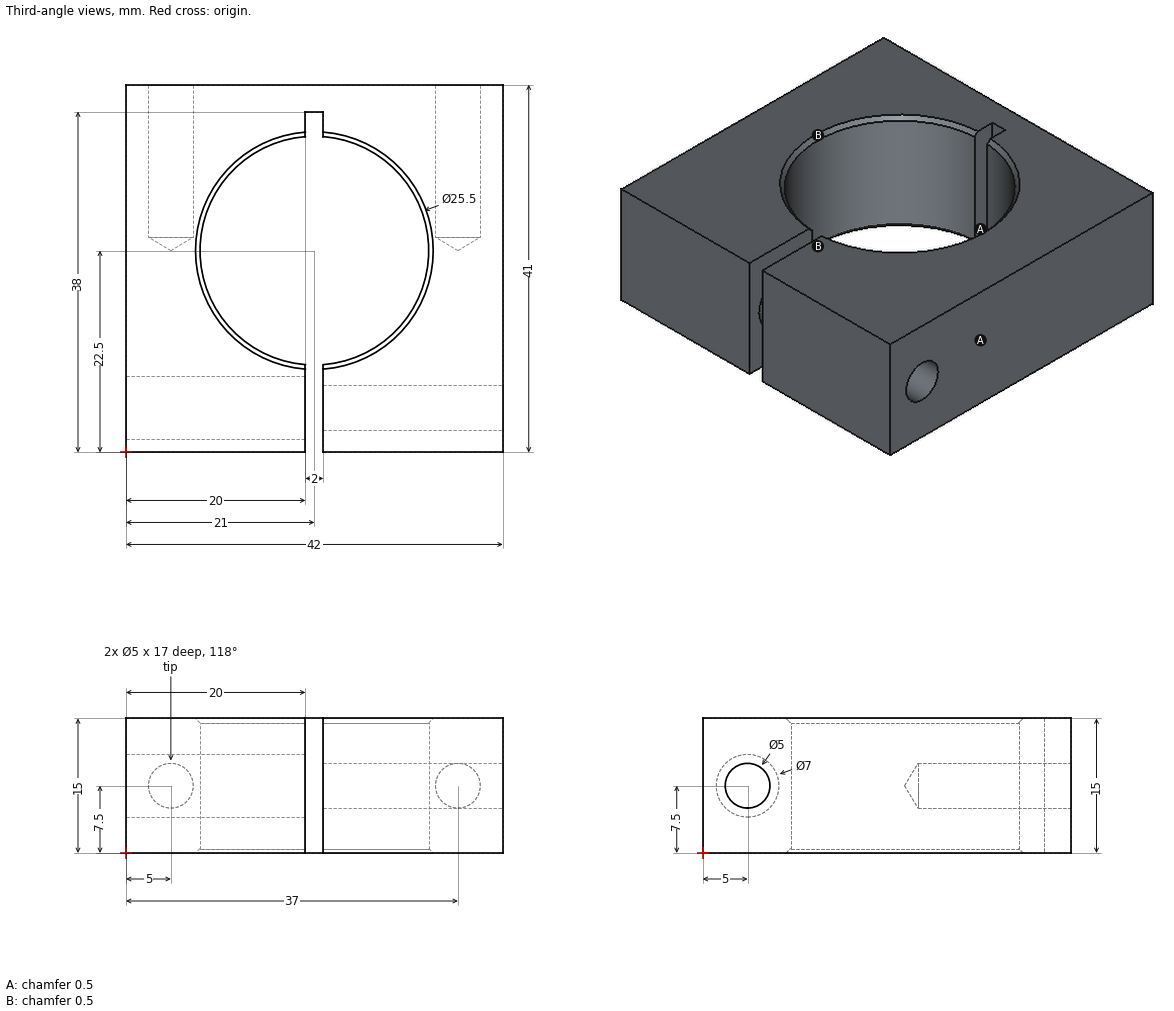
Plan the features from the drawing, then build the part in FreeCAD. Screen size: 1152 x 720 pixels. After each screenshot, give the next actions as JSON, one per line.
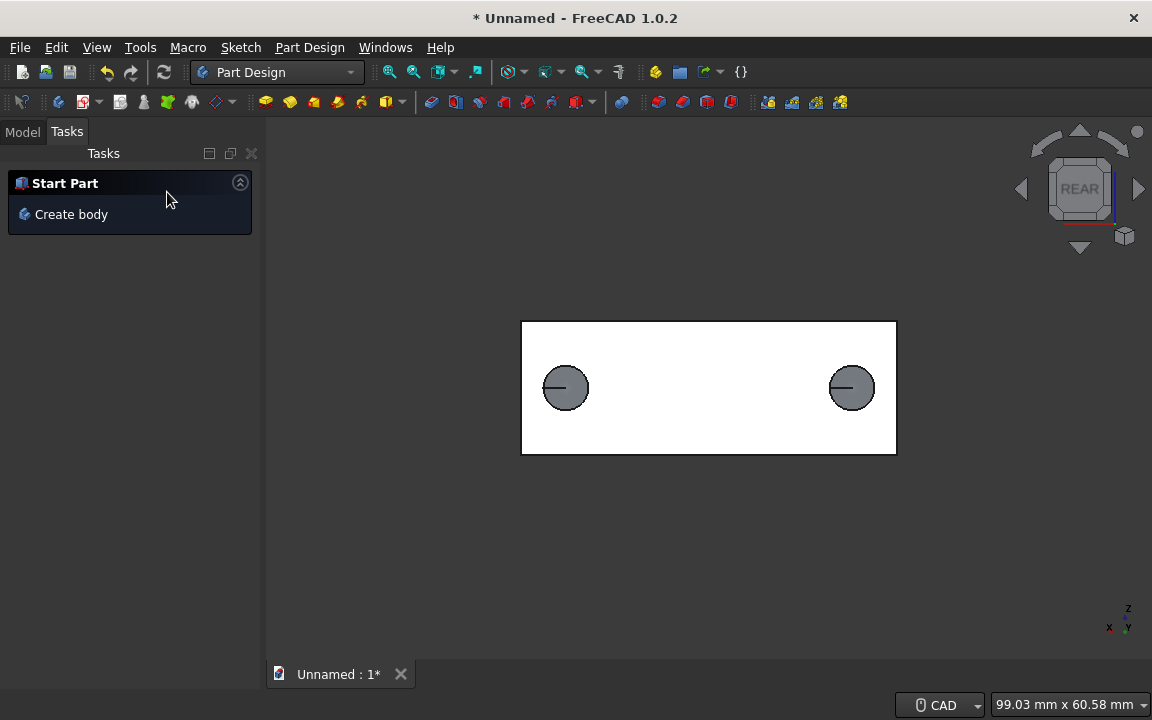
{"action": "left_click", "coordinate": [390, 72]}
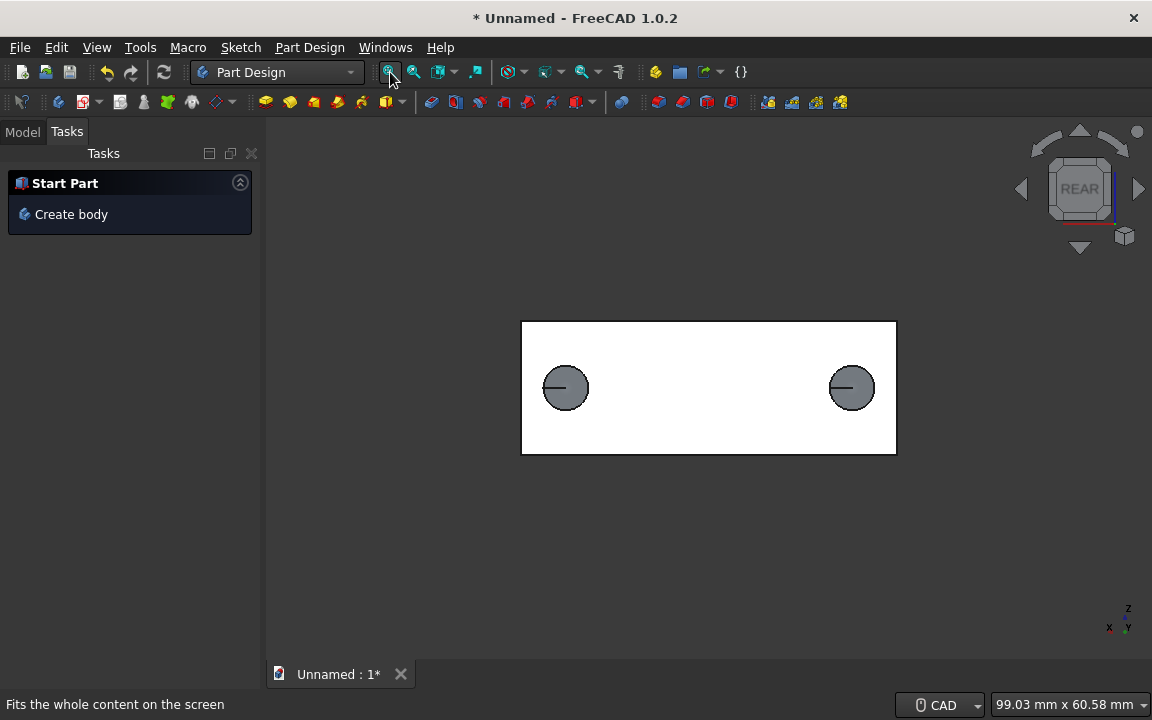
{"action": "key", "text": "6"}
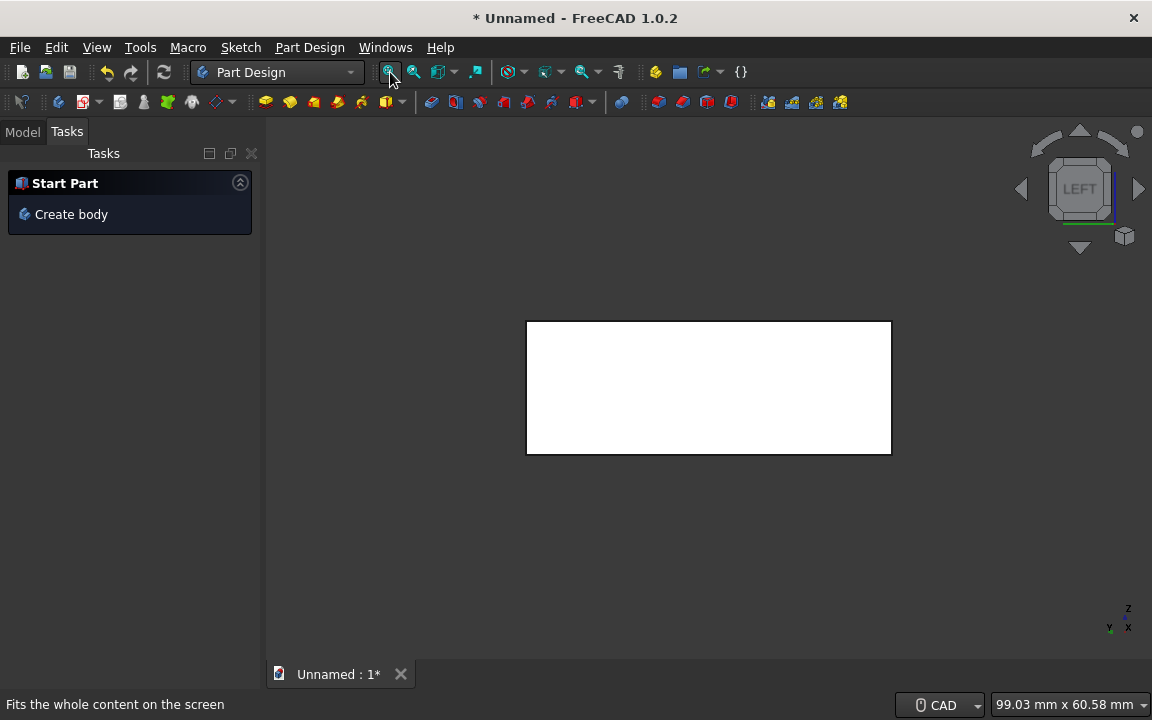
{"action": "left_click", "coordinate": [390, 72]}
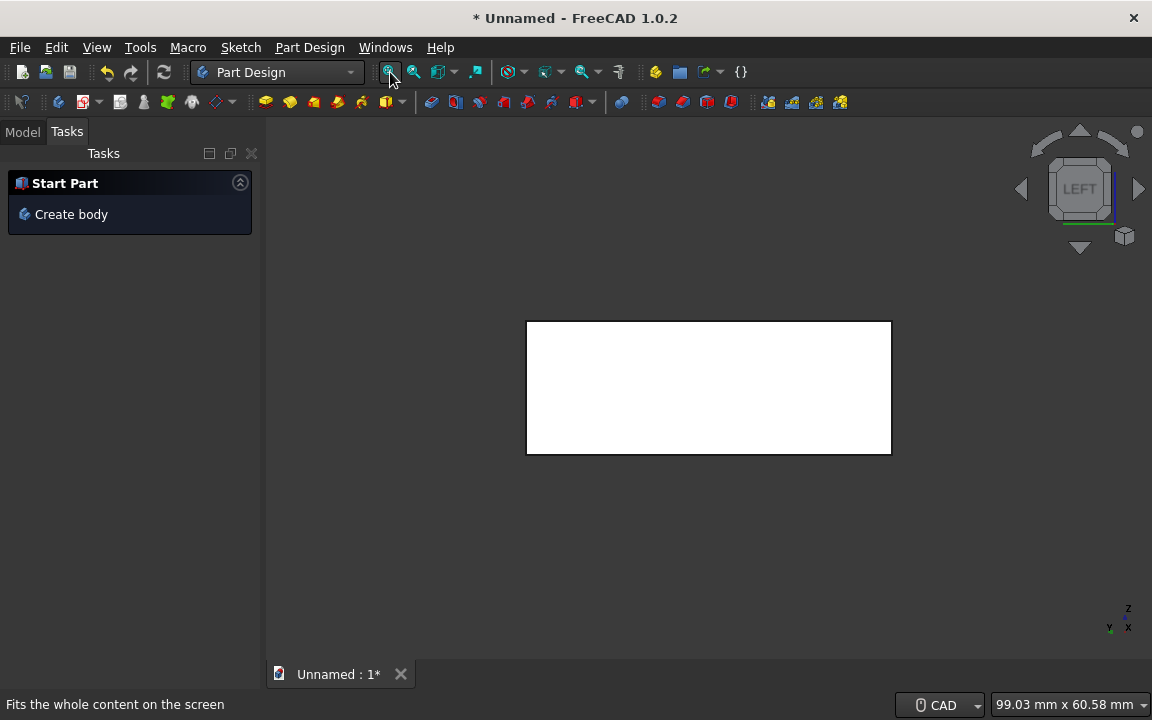
{"action": "left_click", "coordinate": [604, 387]}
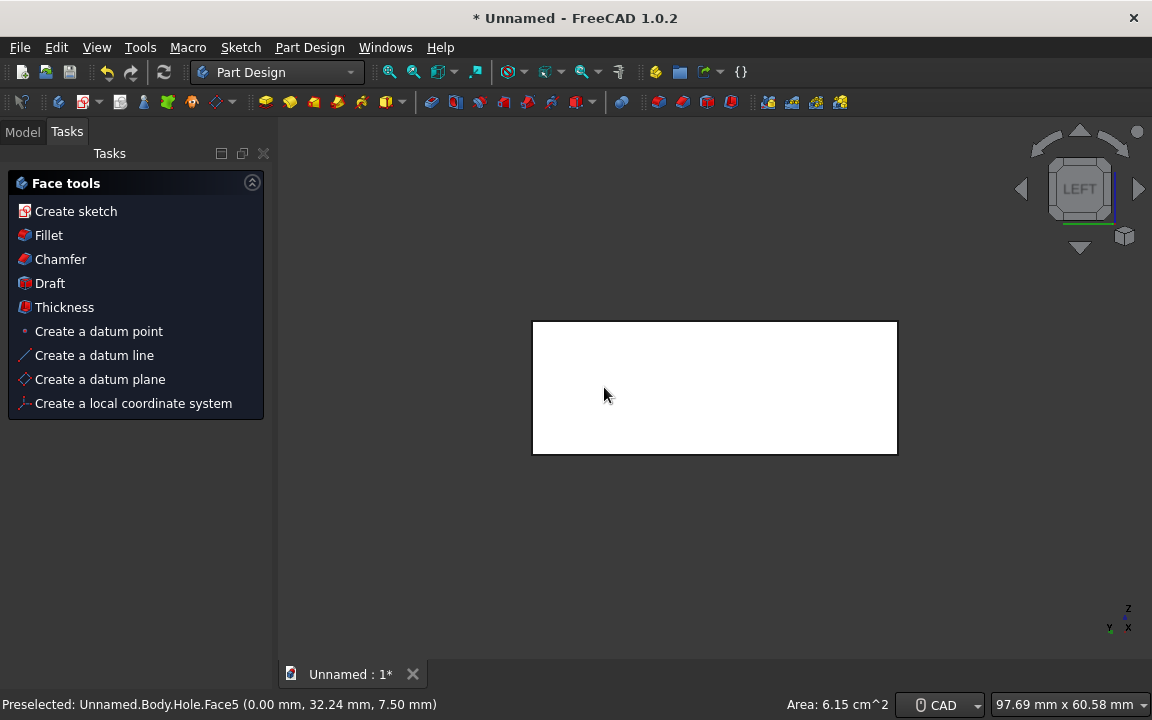
{"action": "left_click", "coordinate": [84, 102]}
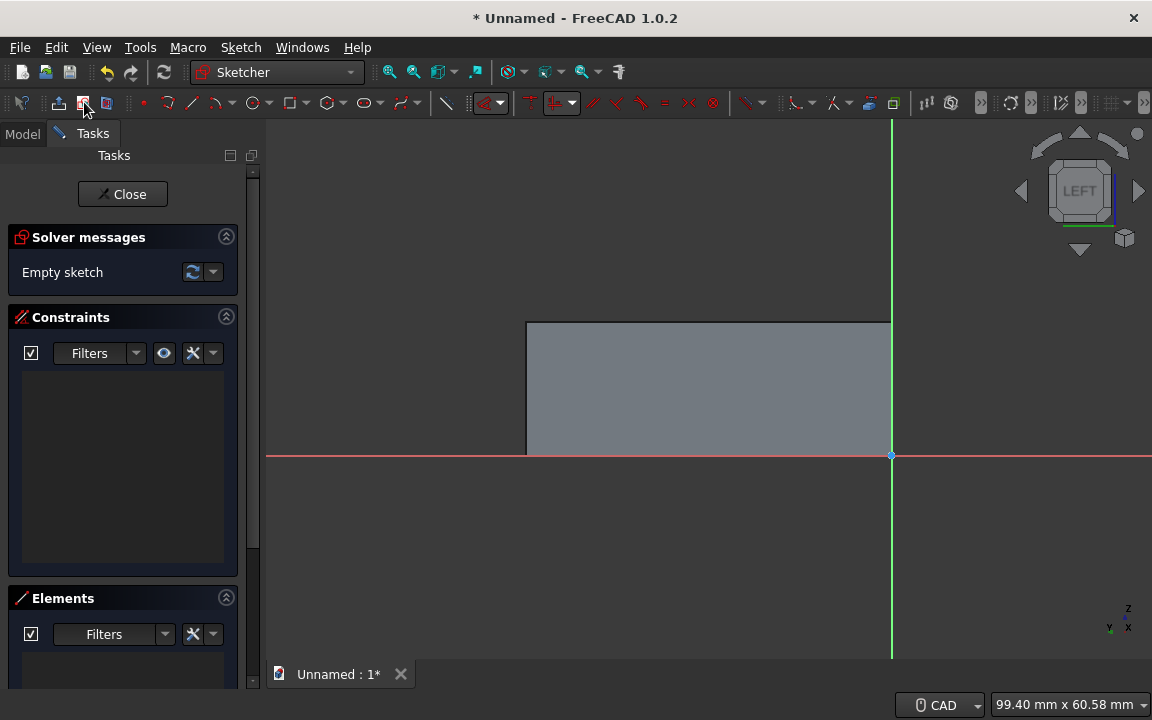
{"action": "scroll", "coordinate": [946, 415], "scroll_direction": "up", "scroll_amount": 6}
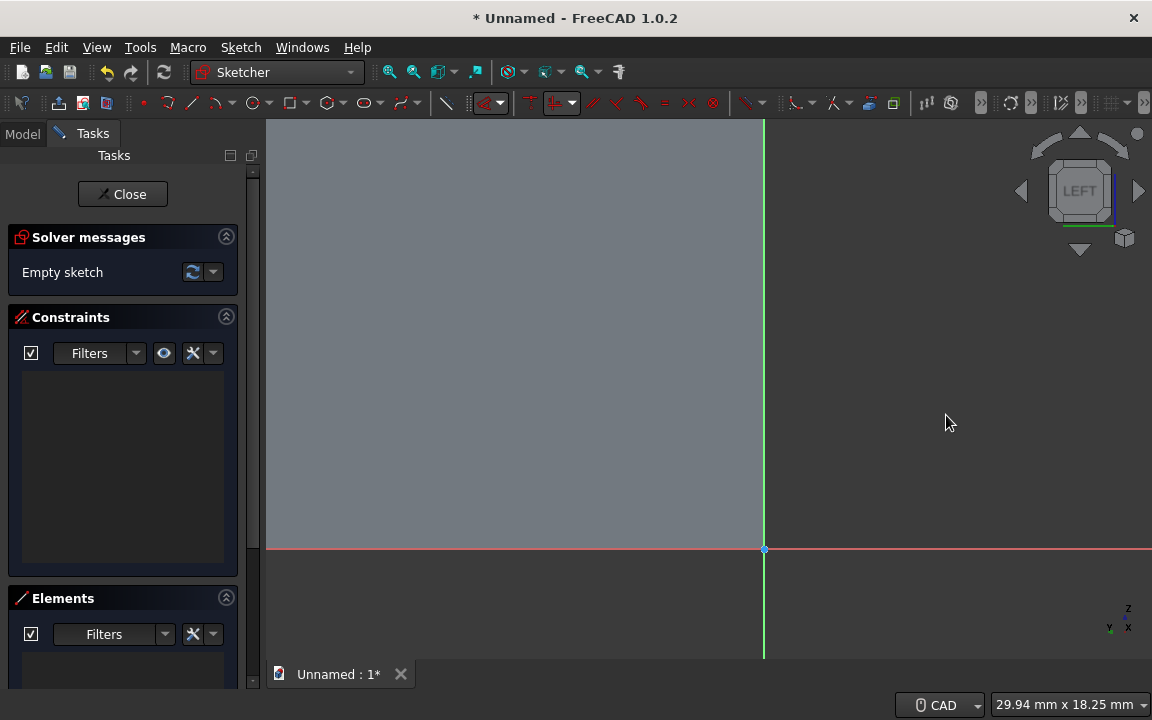
{"action": "left_click", "coordinate": [254, 104]}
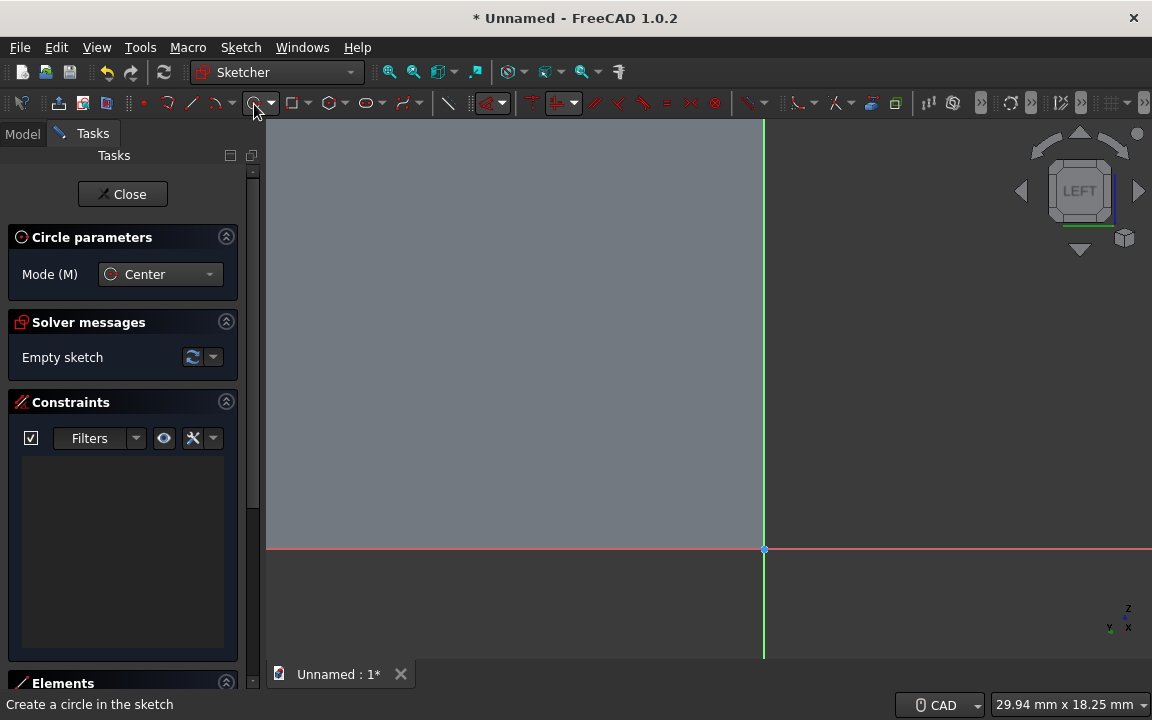
{"action": "left_click", "coordinate": [616, 327]}
{"action": "mouse_move", "coordinate": [689, 254]}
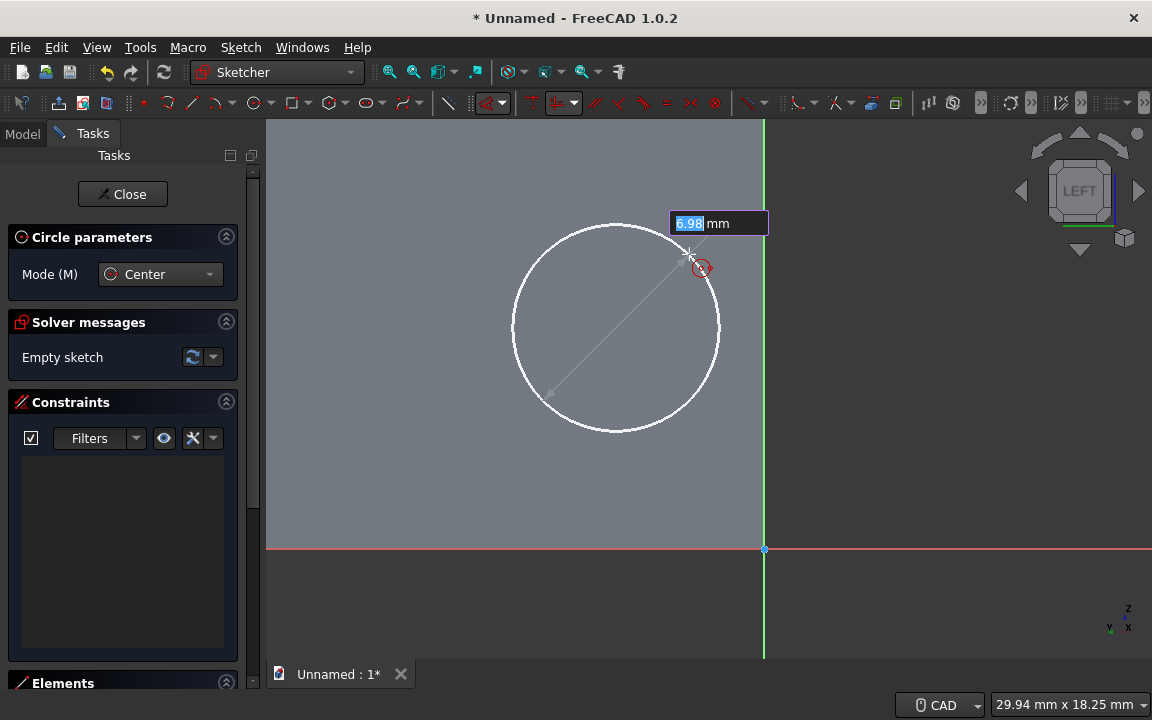
{"action": "type", "text": "7"}
{"action": "key", "text": "Return"}
{"action": "key", "text": "Escape"}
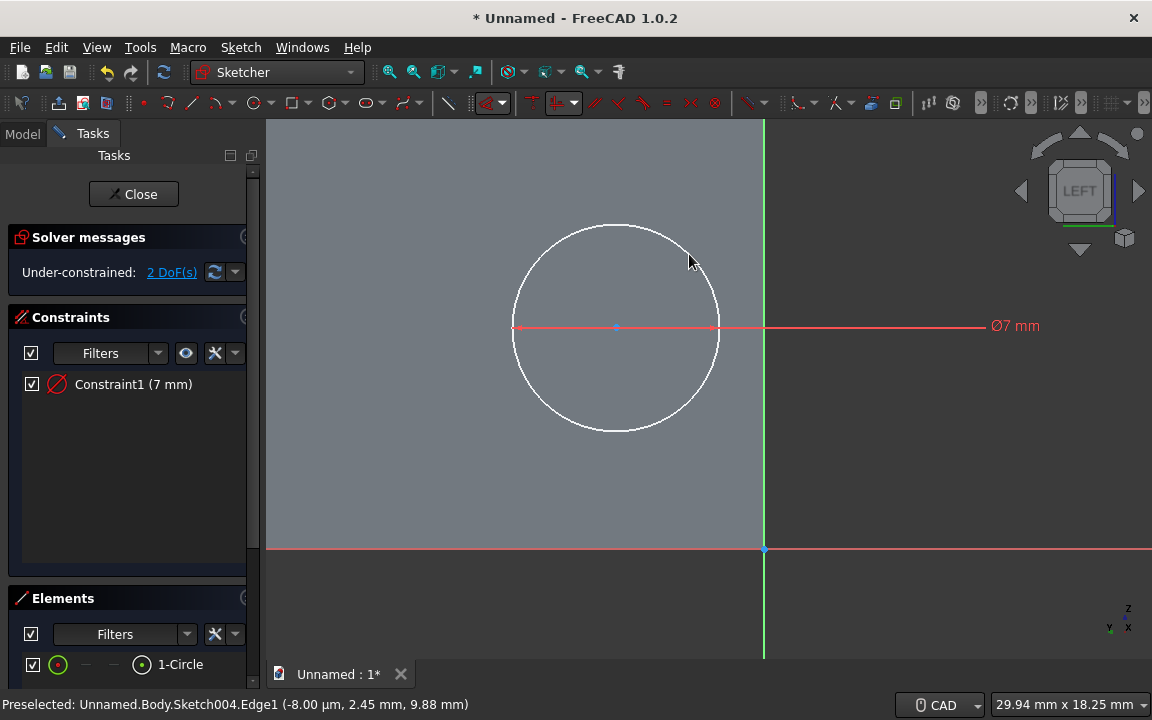
{"action": "left_click", "coordinate": [616, 328]}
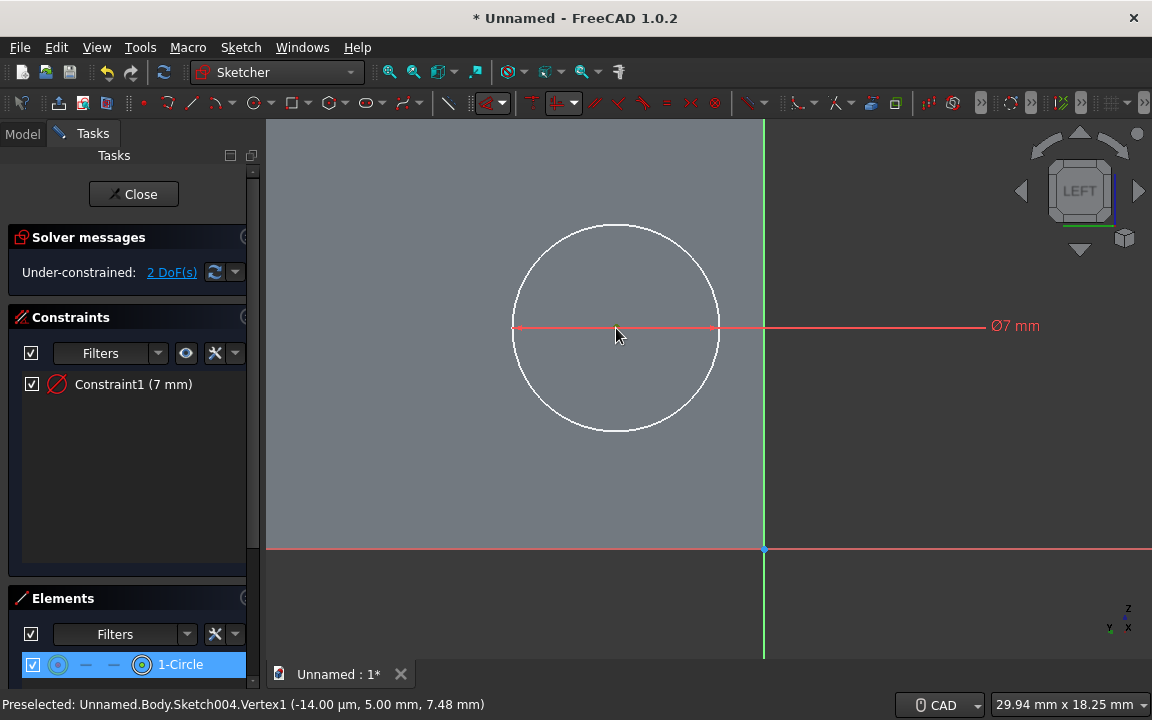
{"action": "left_click", "coordinate": [504, 104]}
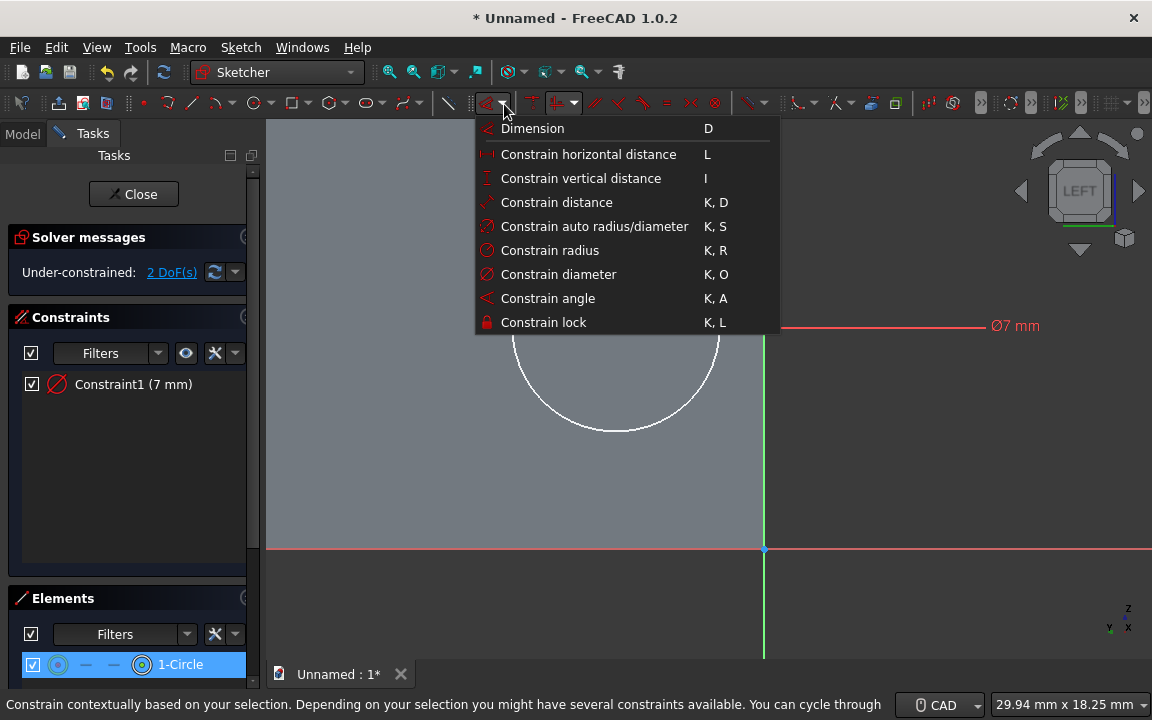
{"action": "left_click", "coordinate": [628, 154]}